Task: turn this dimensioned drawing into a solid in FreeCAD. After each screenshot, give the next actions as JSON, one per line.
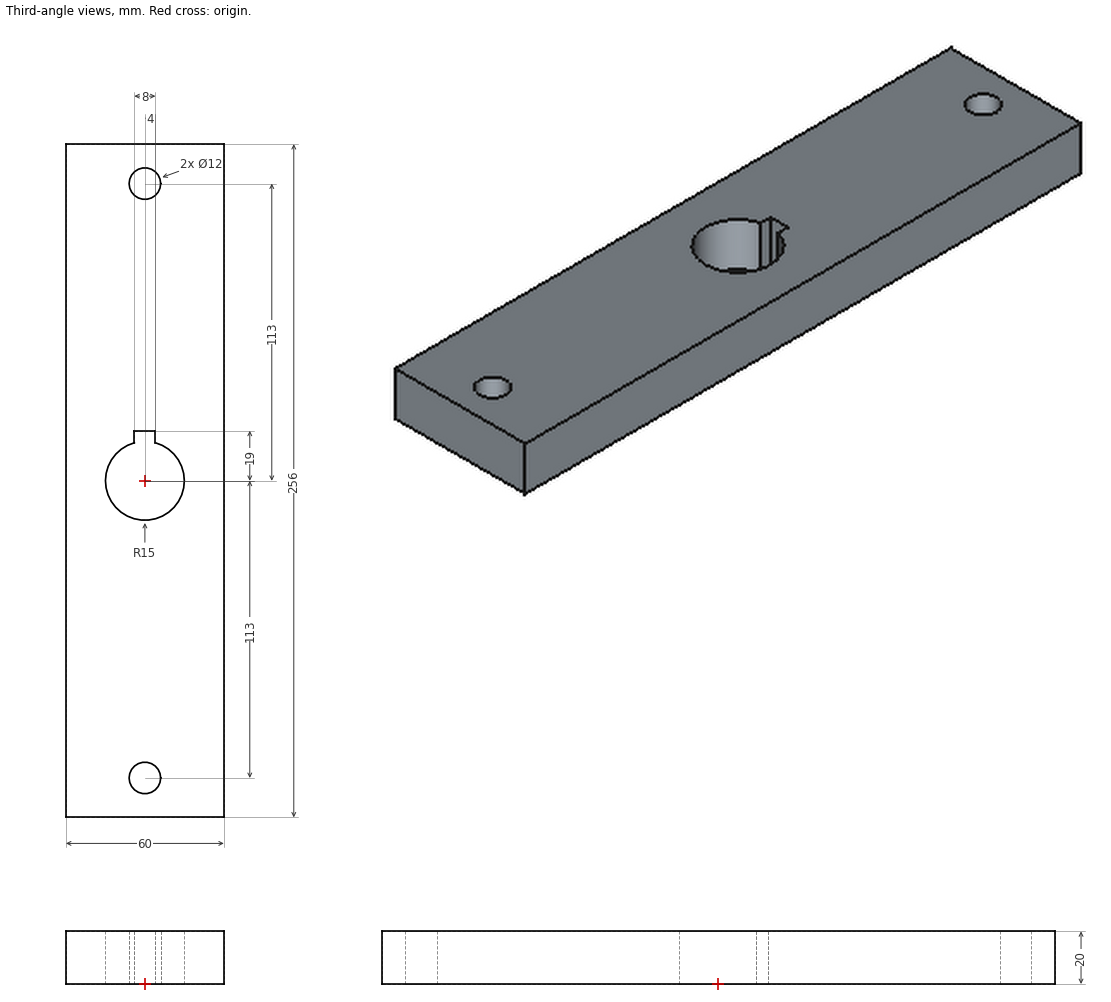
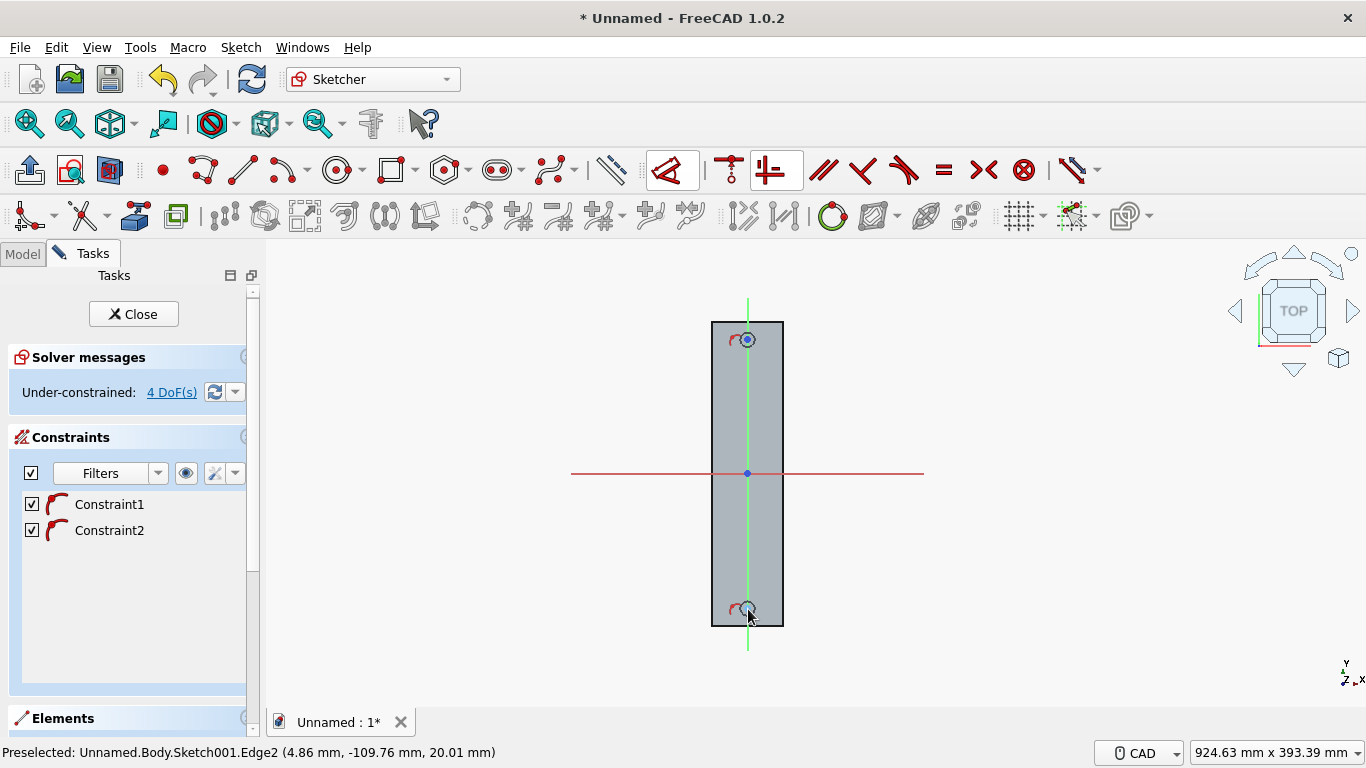
{"action": "scroll", "coordinate": [753, 335], "scroll_direction": "up", "scroll_amount": 6}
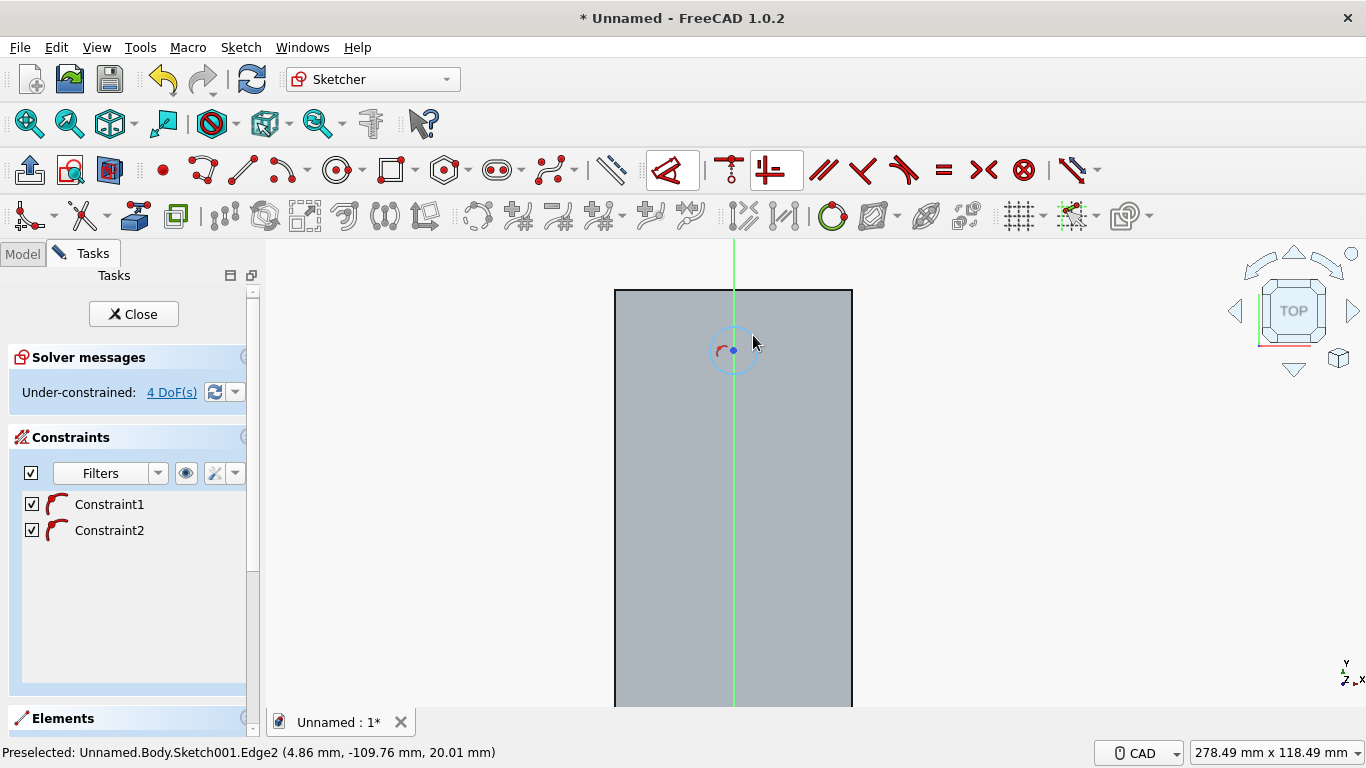
{"action": "left_click", "coordinate": [751, 334]}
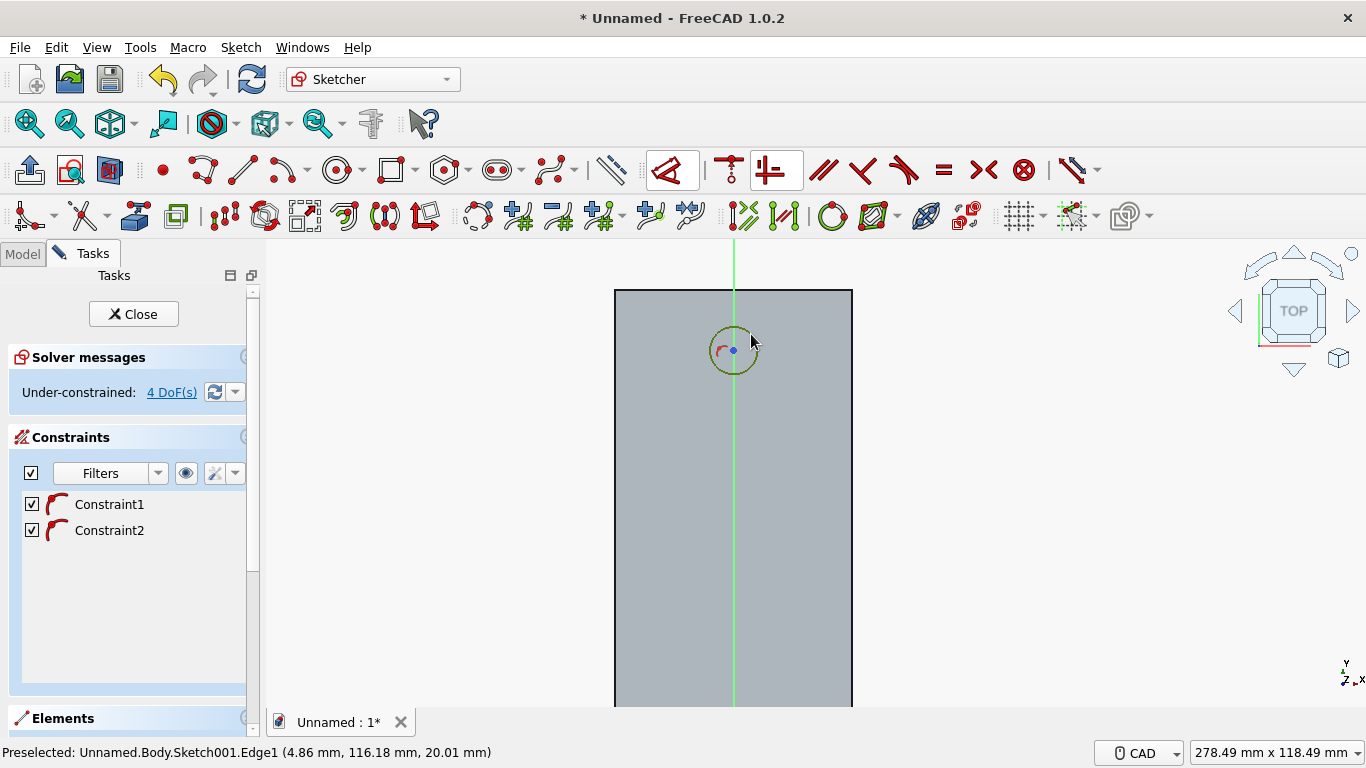
{"action": "scroll", "coordinate": [753, 334], "scroll_direction": "down", "scroll_amount": 6}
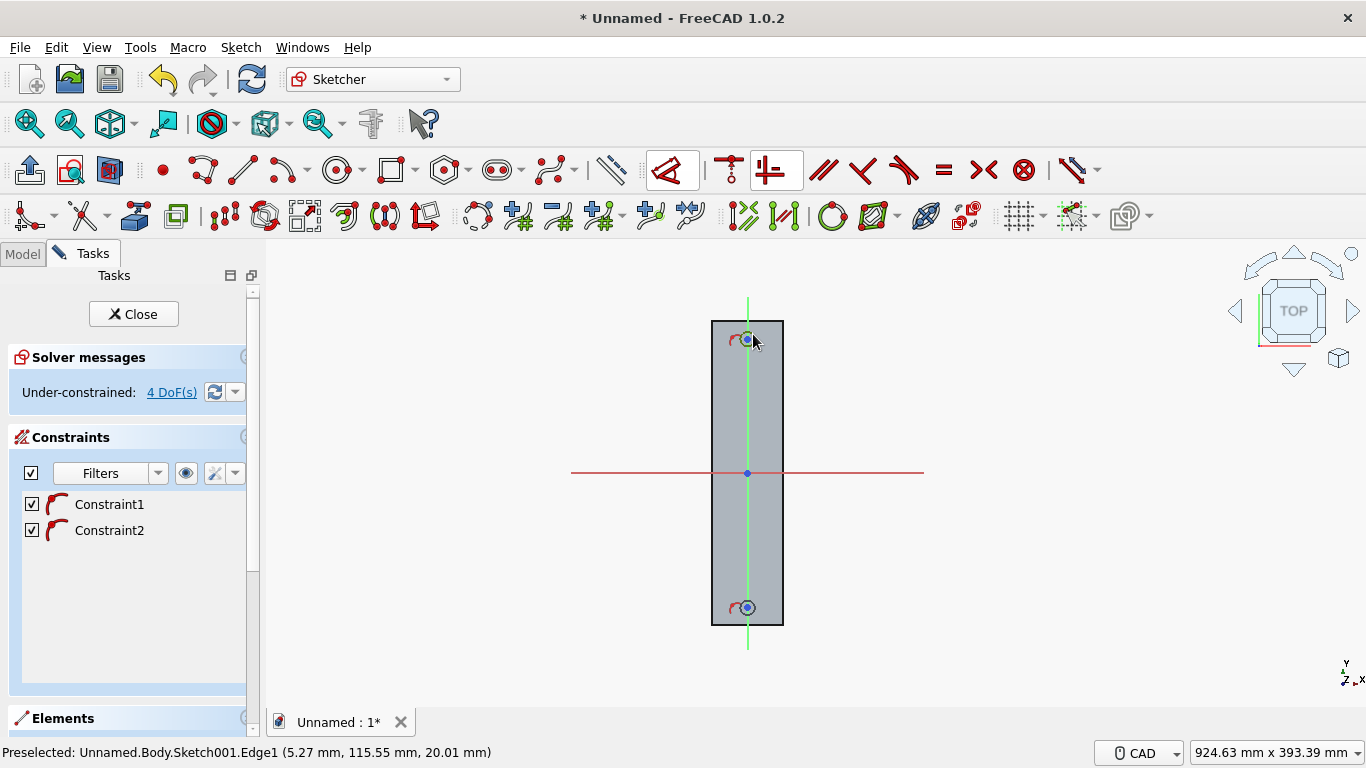
{"action": "scroll", "coordinate": [753, 603], "scroll_direction": "up", "scroll_amount": 6}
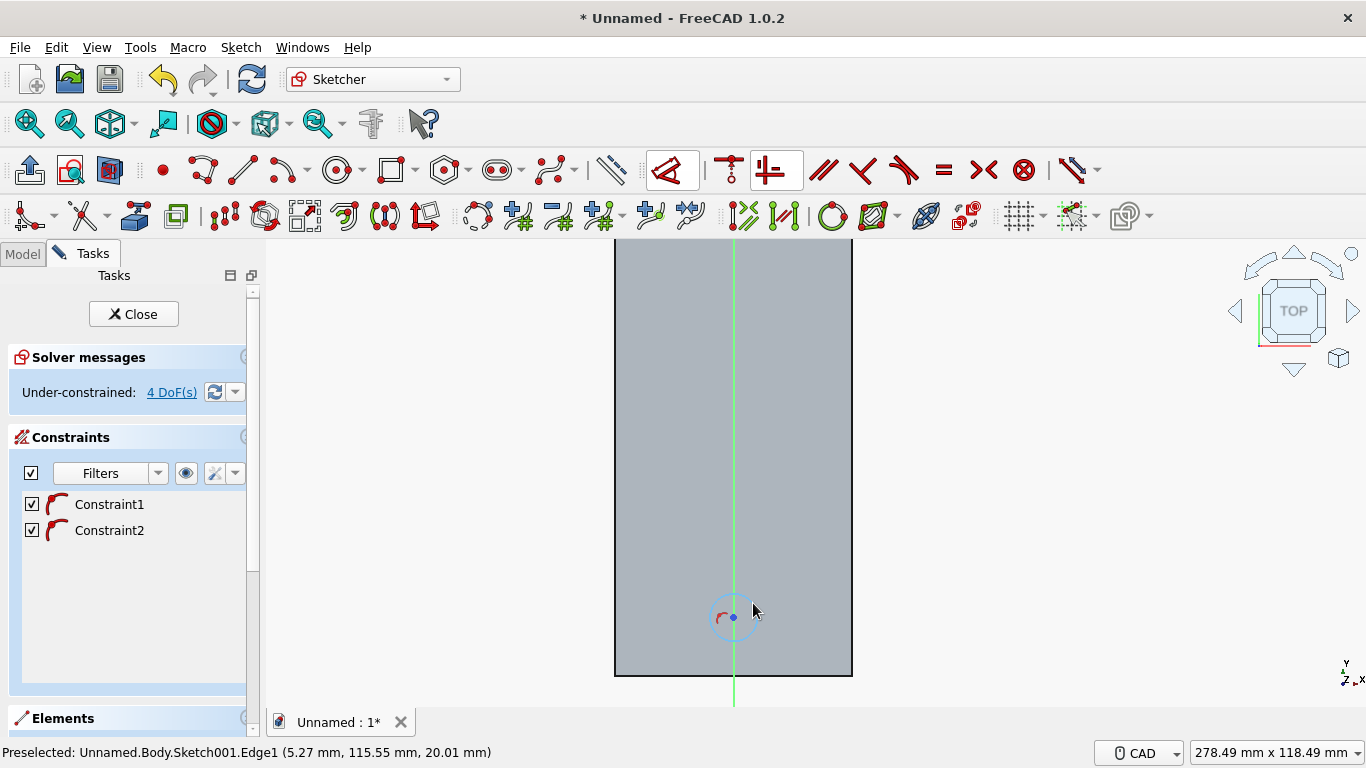
{"action": "left_click", "coordinate": [751, 601]}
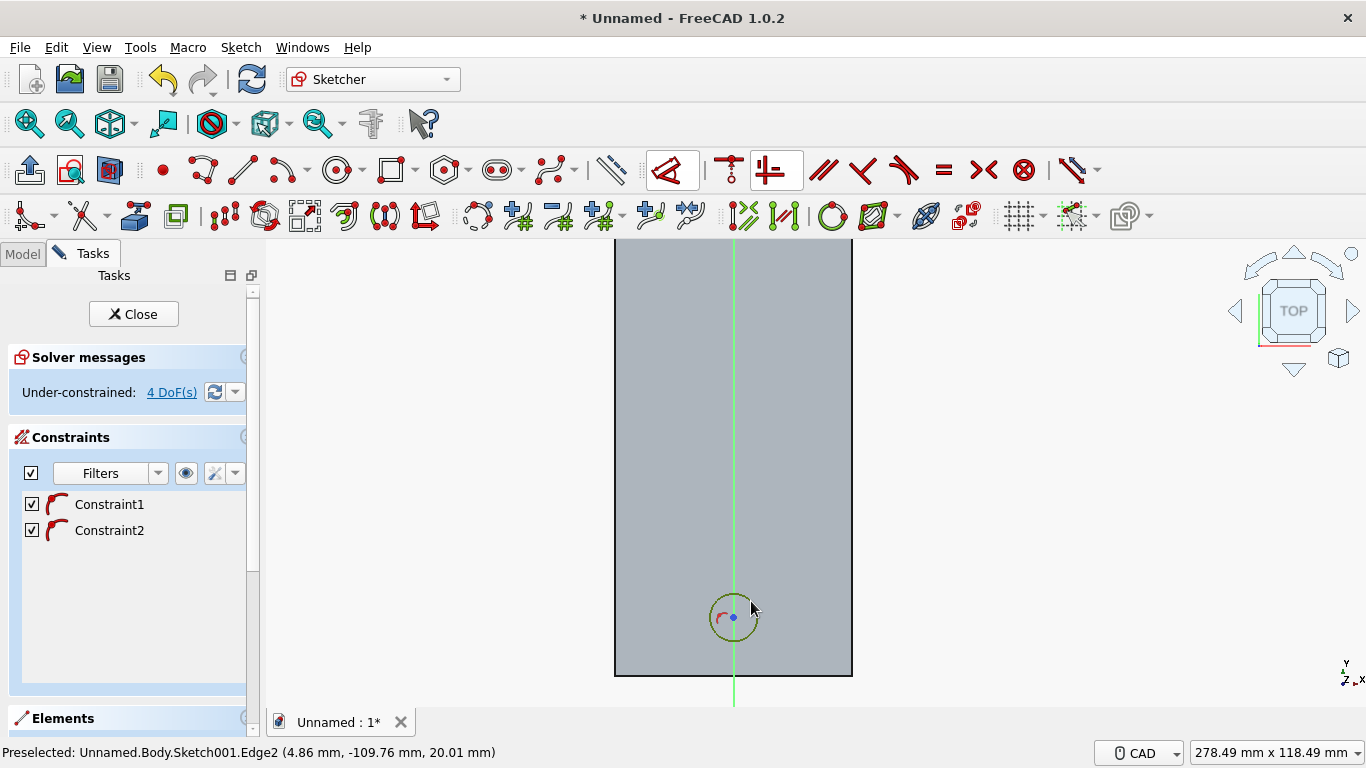
{"action": "key", "text": "e"}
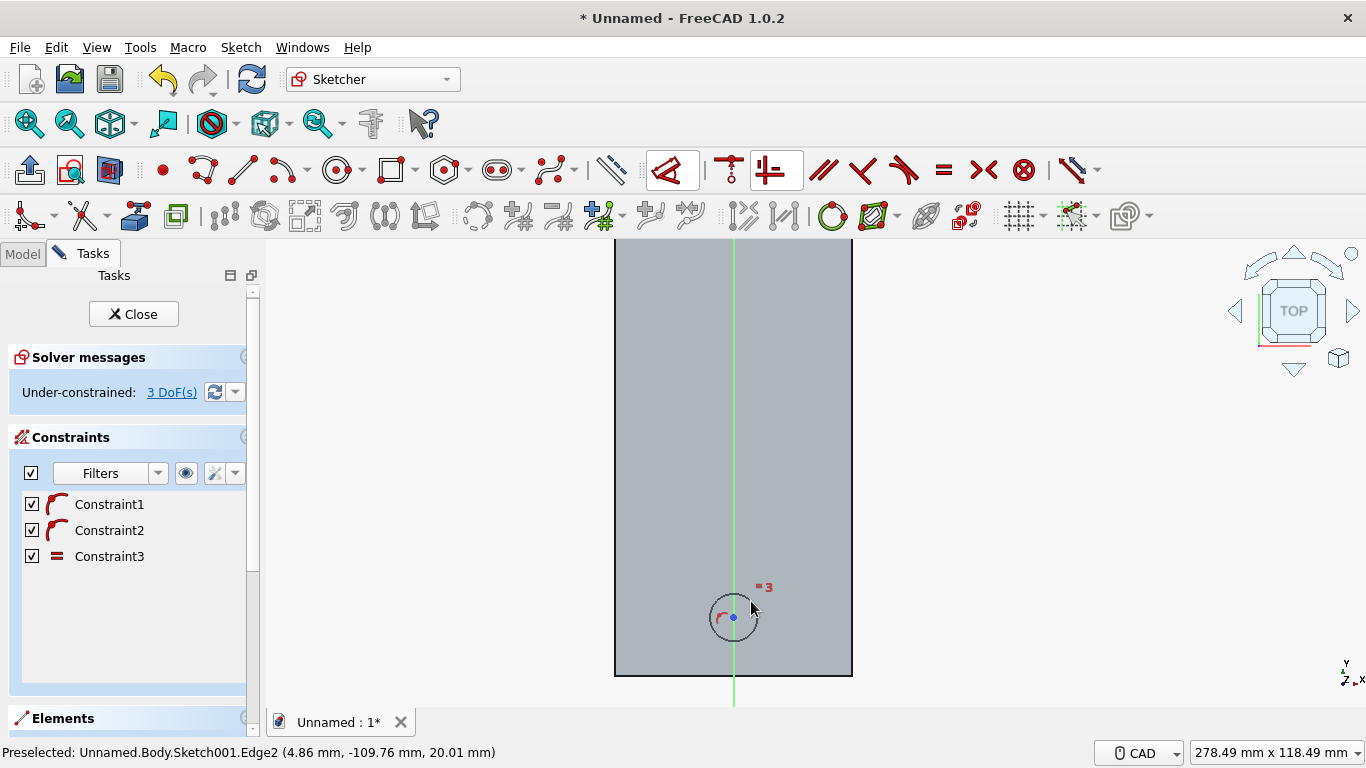
{"action": "left_click", "coordinate": [666, 170]}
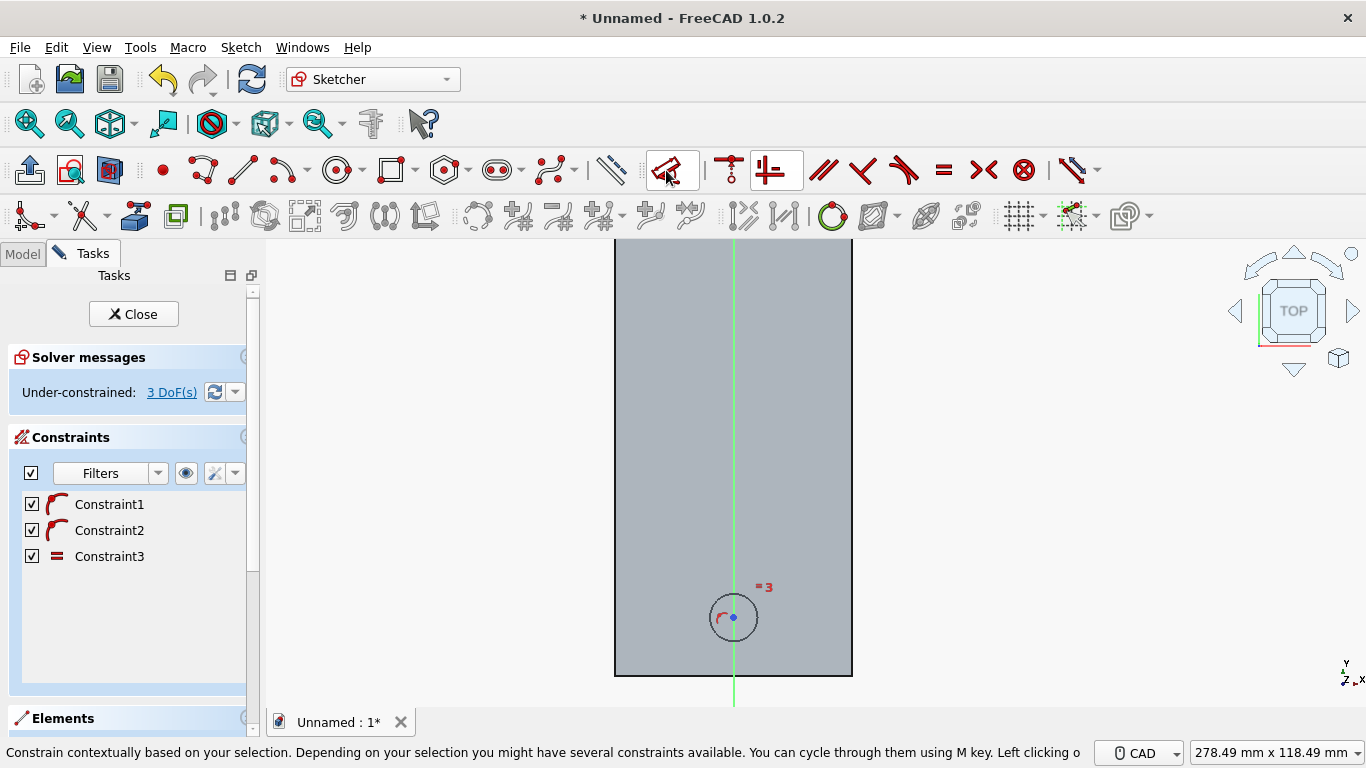
{"action": "scroll", "coordinate": [753, 604], "scroll_direction": "down", "scroll_amount": 6}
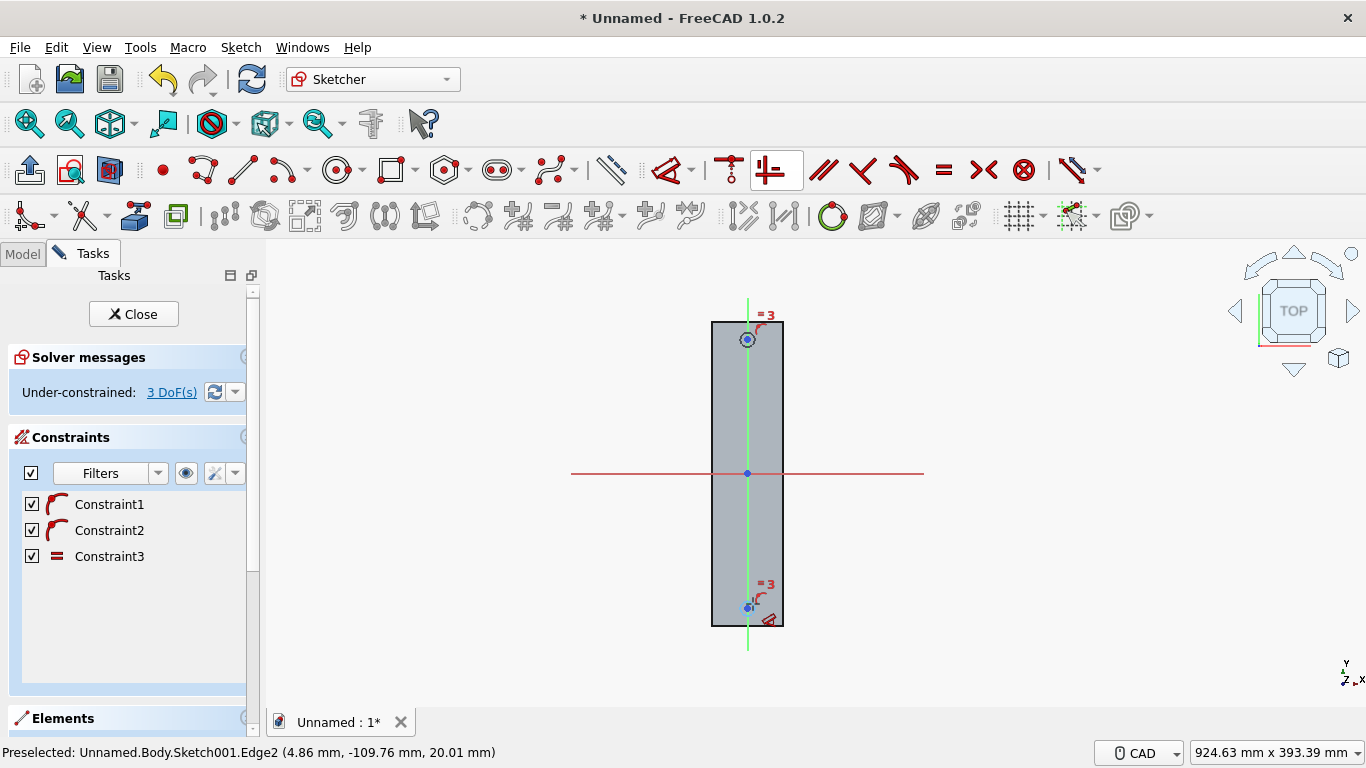
{"action": "scroll", "coordinate": [753, 335], "scroll_direction": "up", "scroll_amount": 6}